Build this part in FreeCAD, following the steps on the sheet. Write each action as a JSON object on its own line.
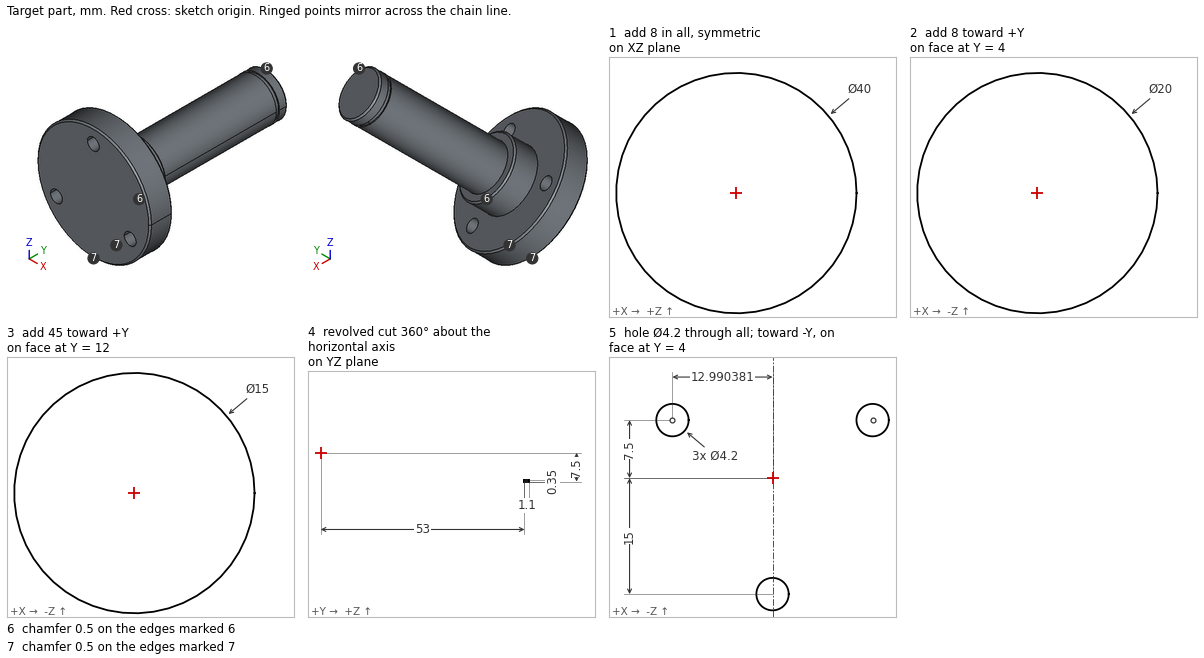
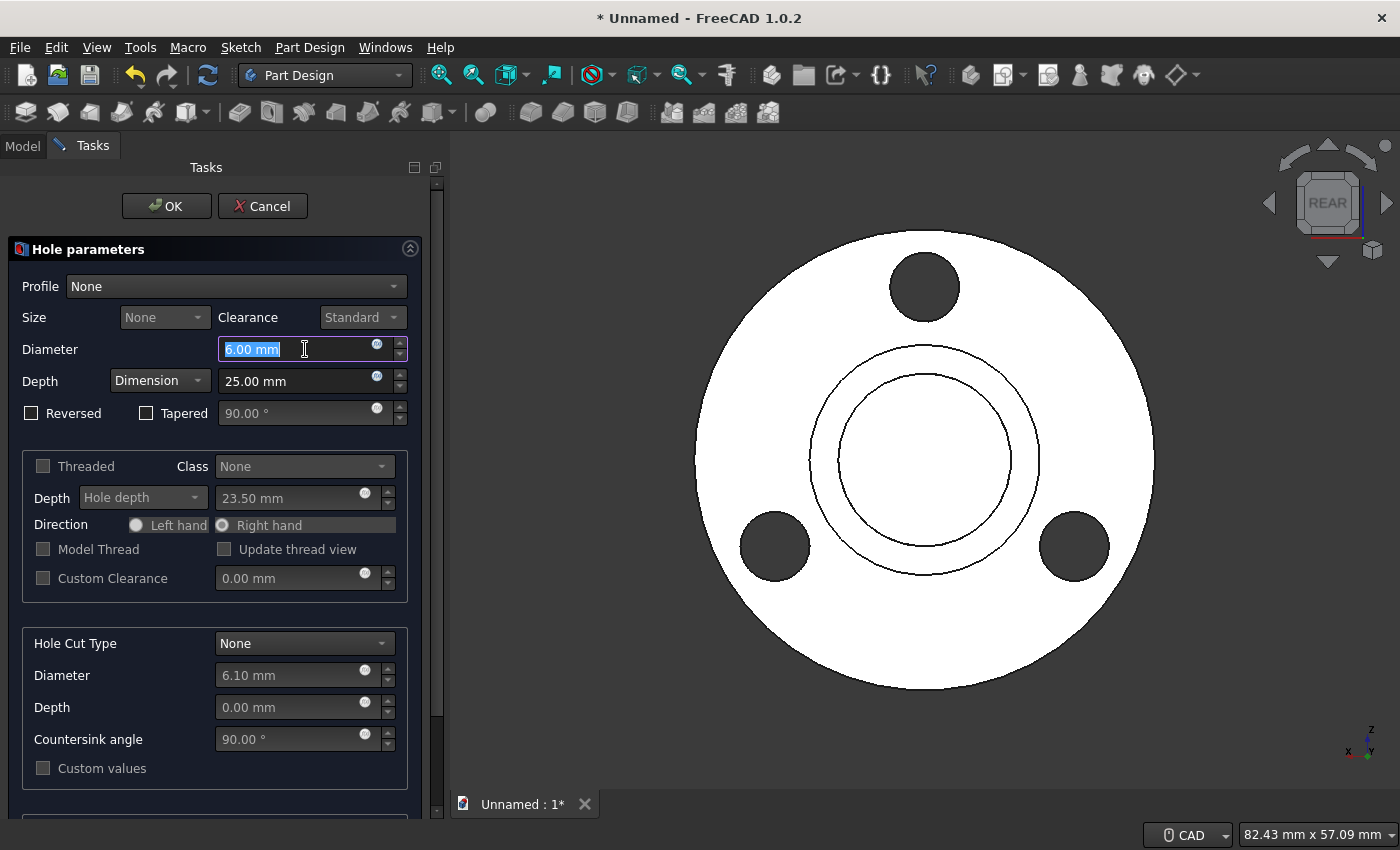
{"action": "type", "text": "4.2"}
{"action": "key", "text": "Tab"}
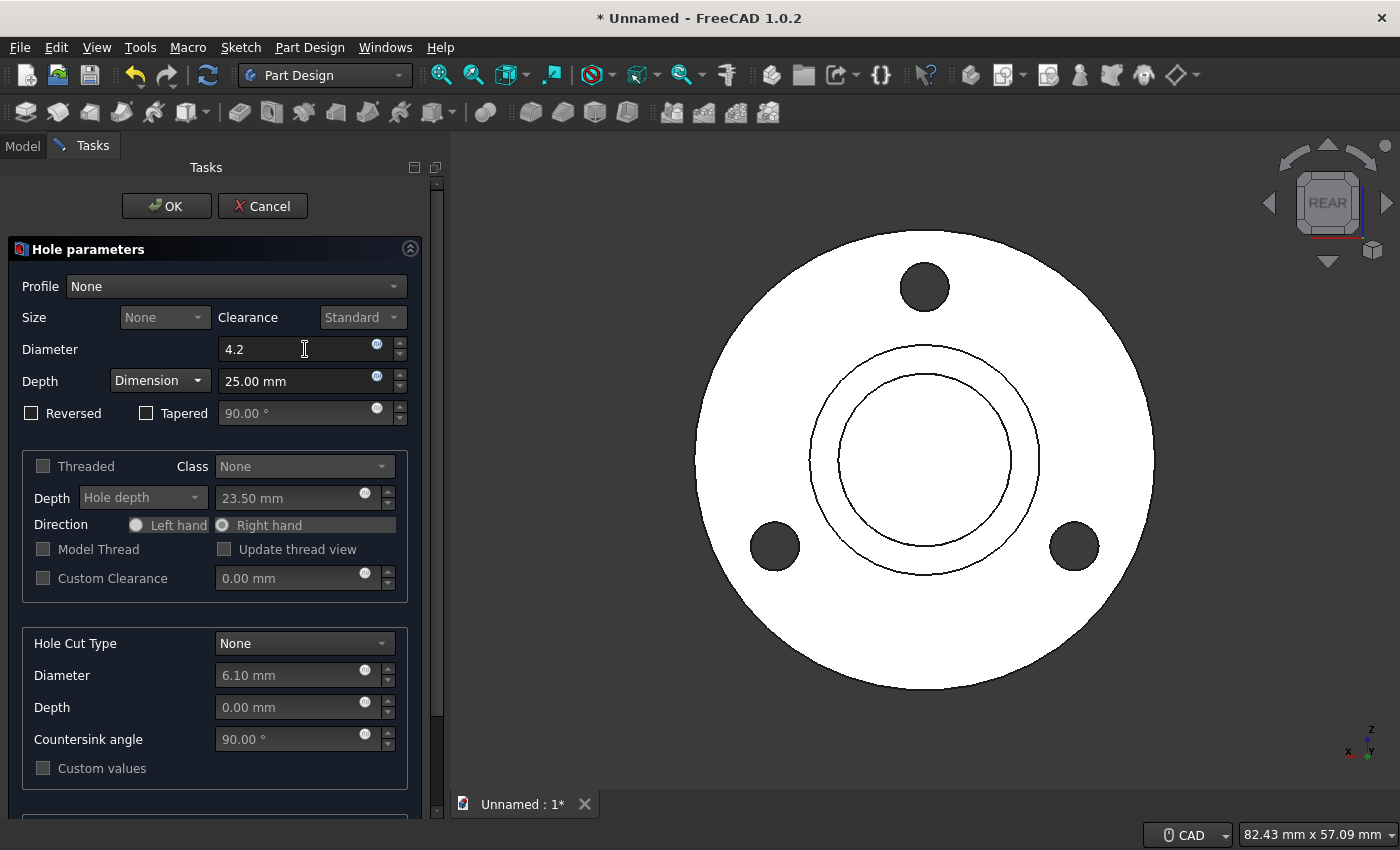
{"action": "left_click", "coordinate": [161, 380]}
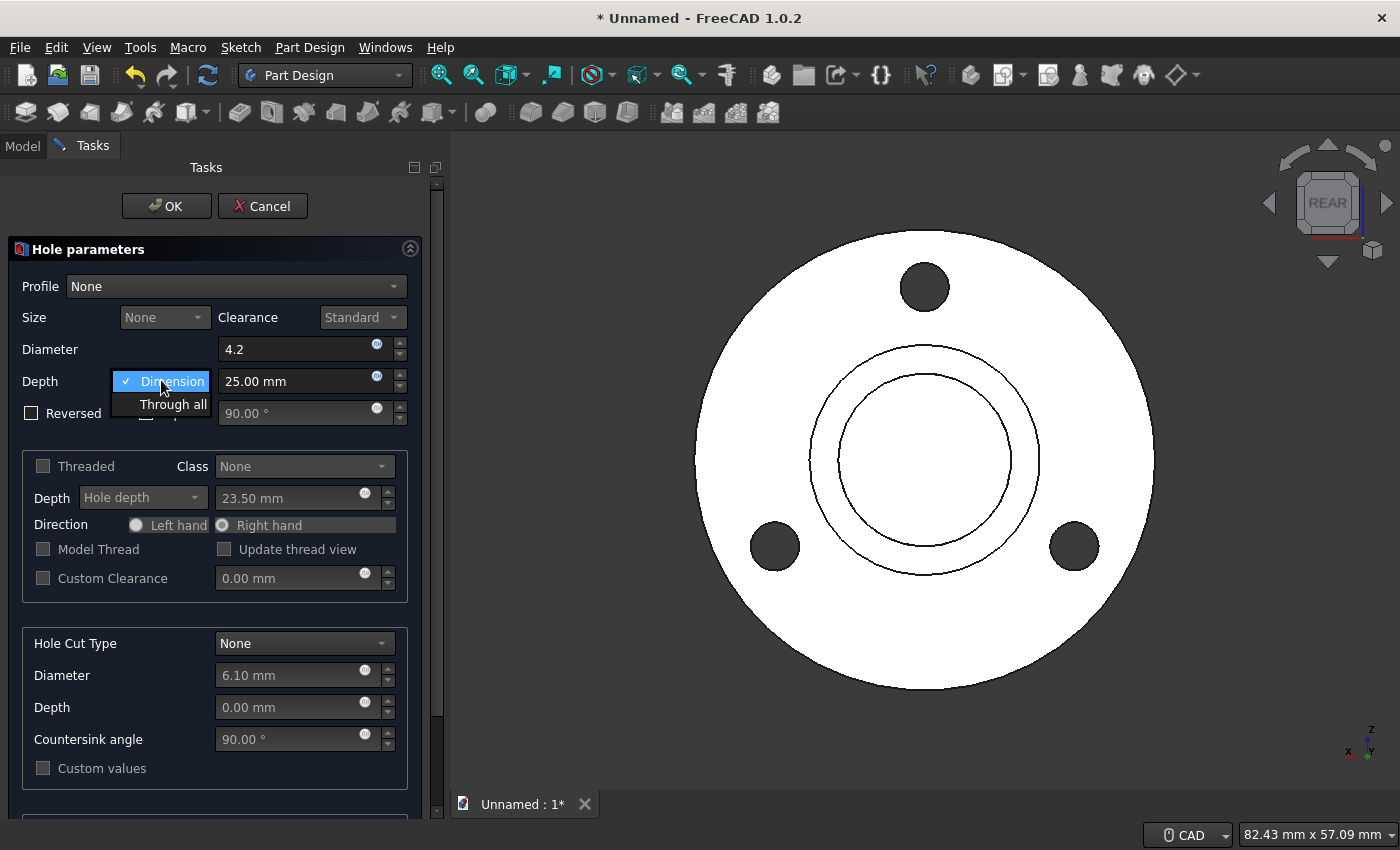
{"action": "left_click", "coordinate": [160, 404]}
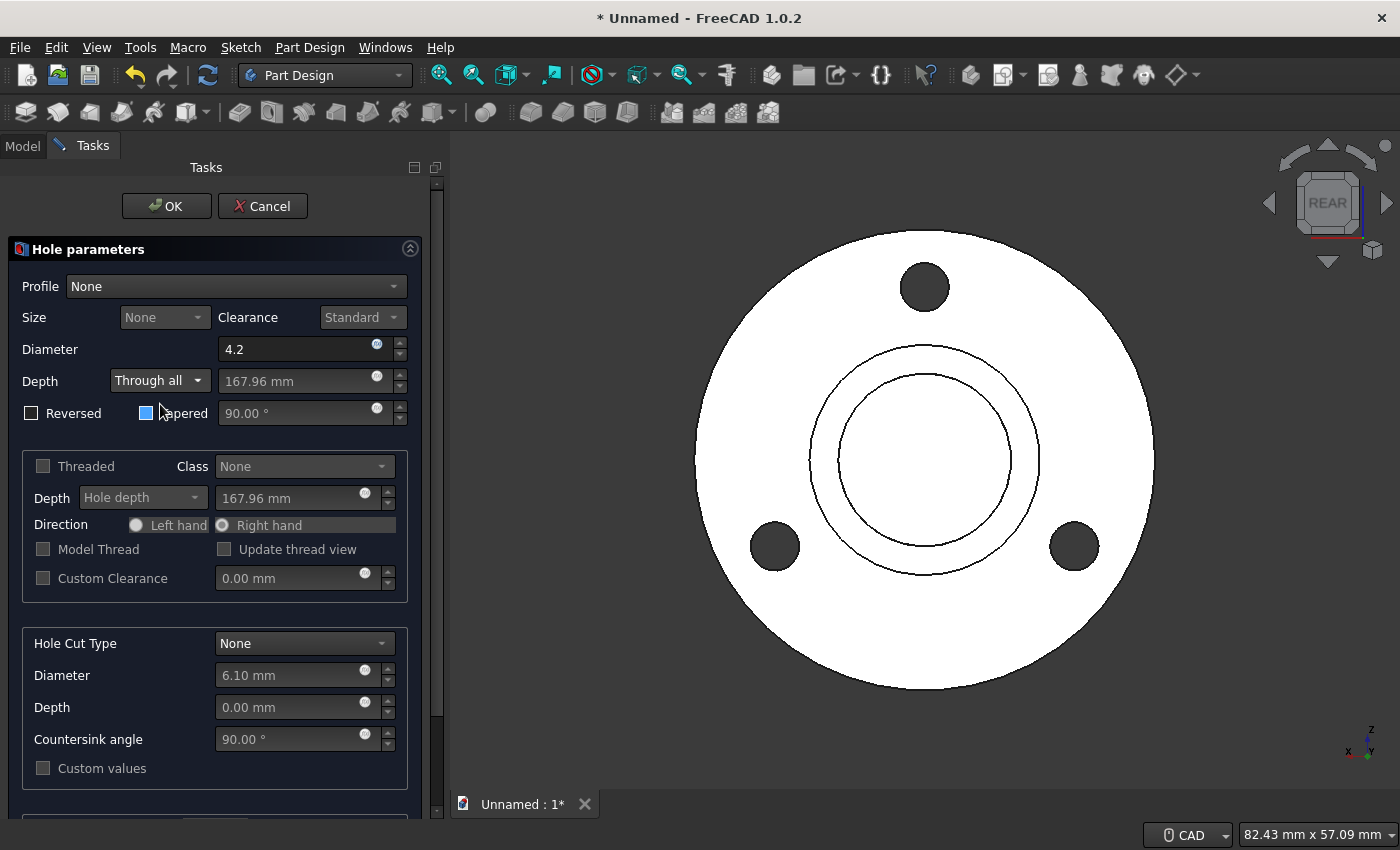
{"action": "left_click", "coordinate": [167, 206]}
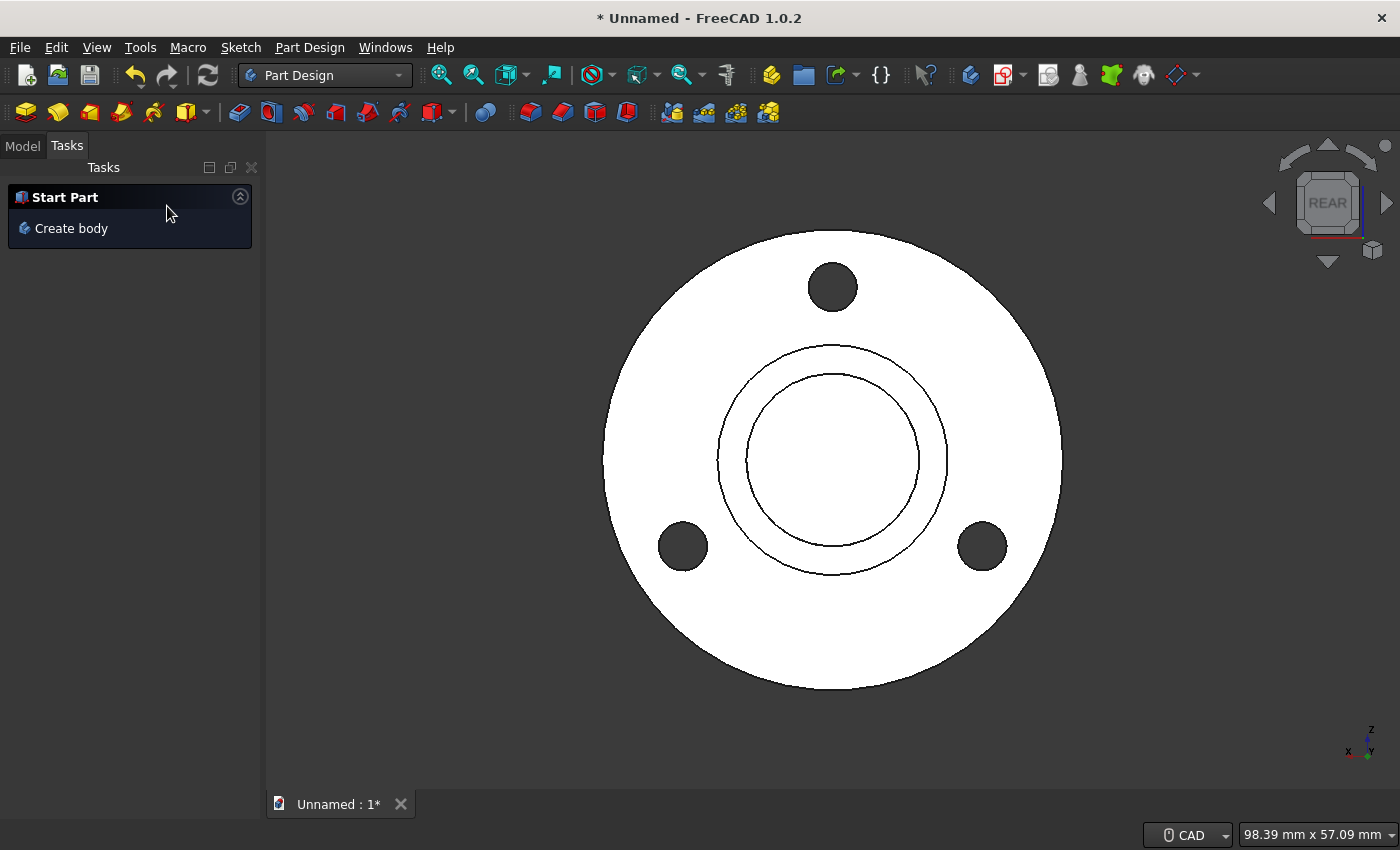
{"action": "left_click", "coordinate": [919, 459]}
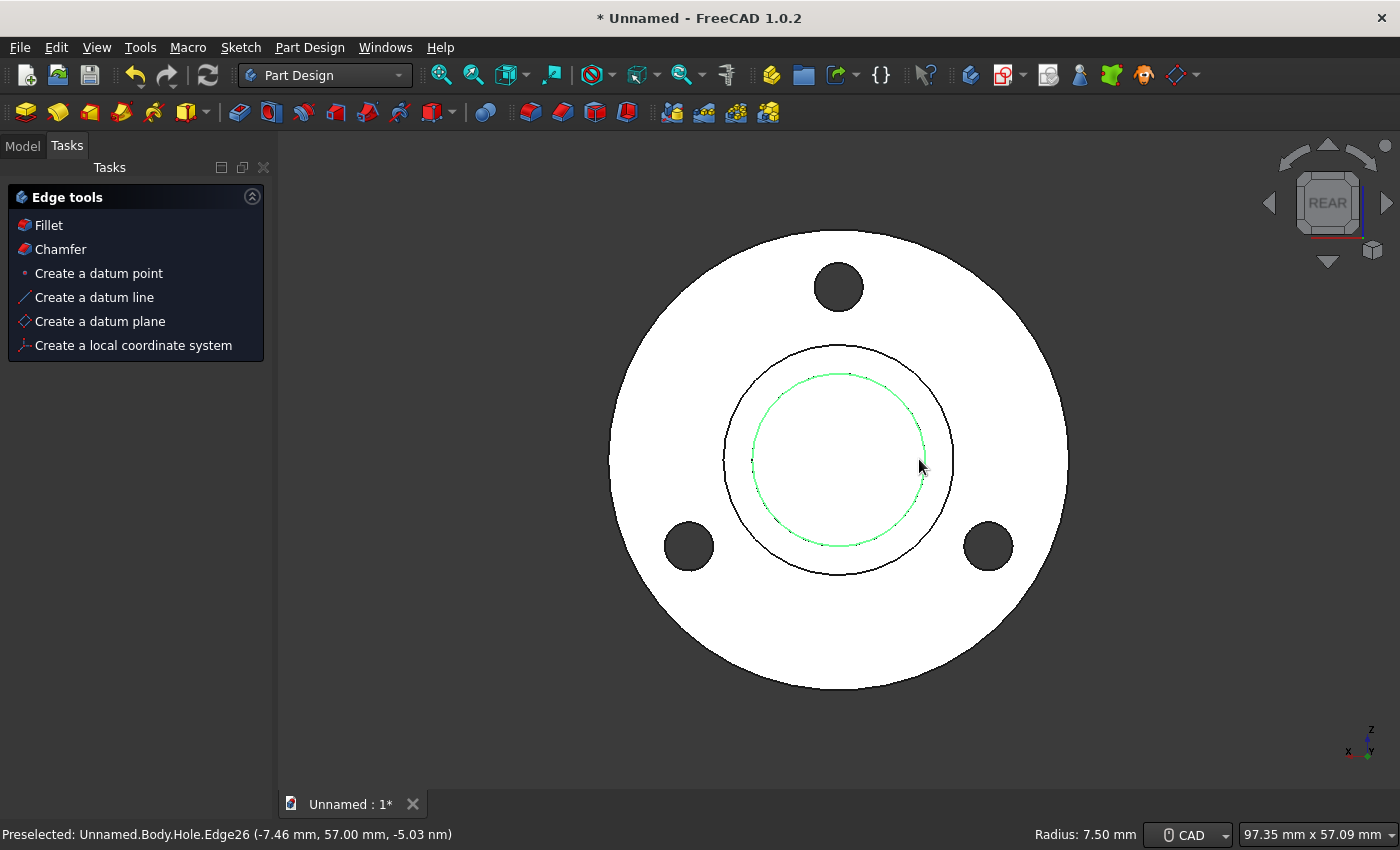
{"action": "left_click", "coordinate": [954, 459], "text": "ctrl"}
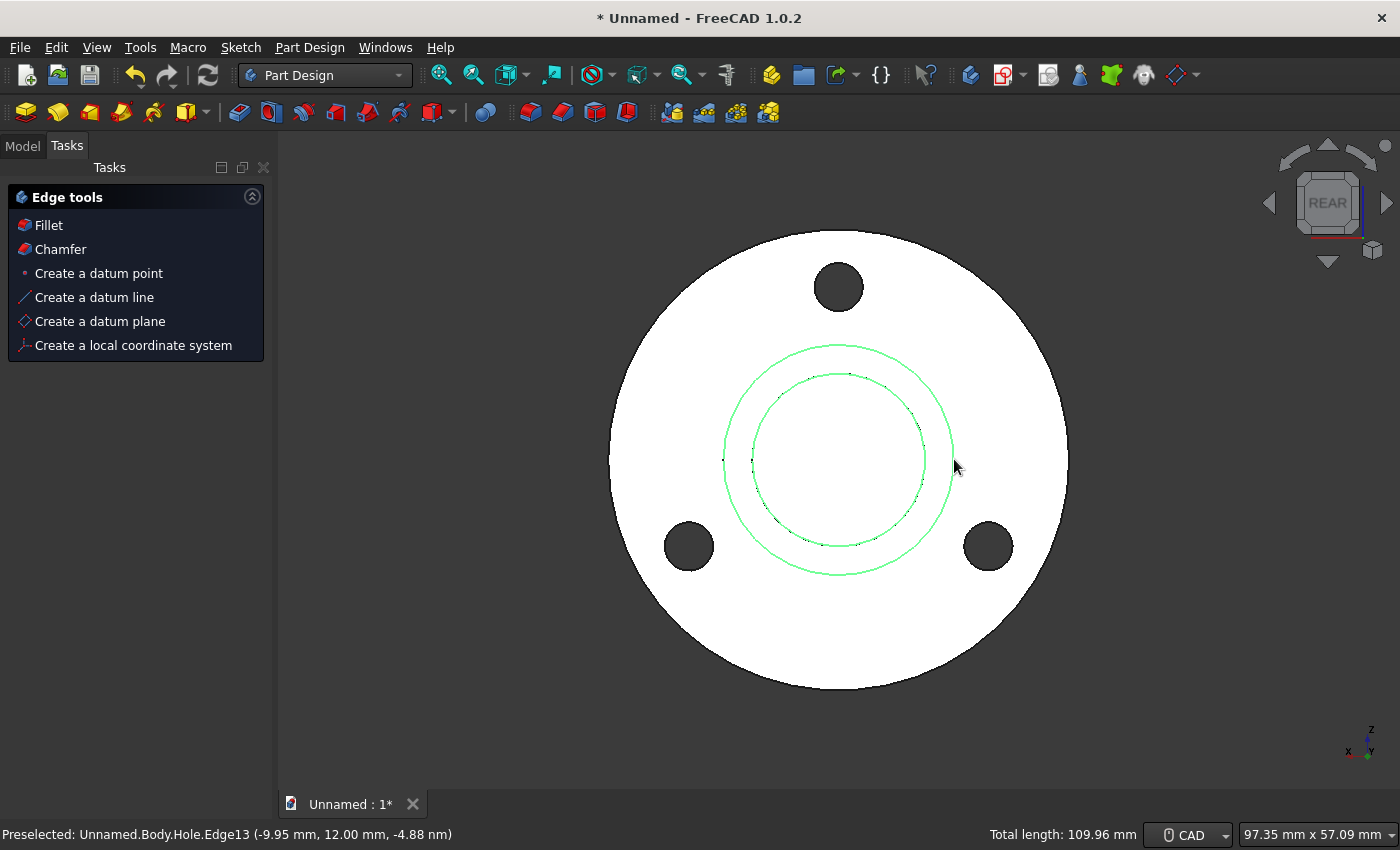
{"action": "left_click", "coordinate": [564, 112]}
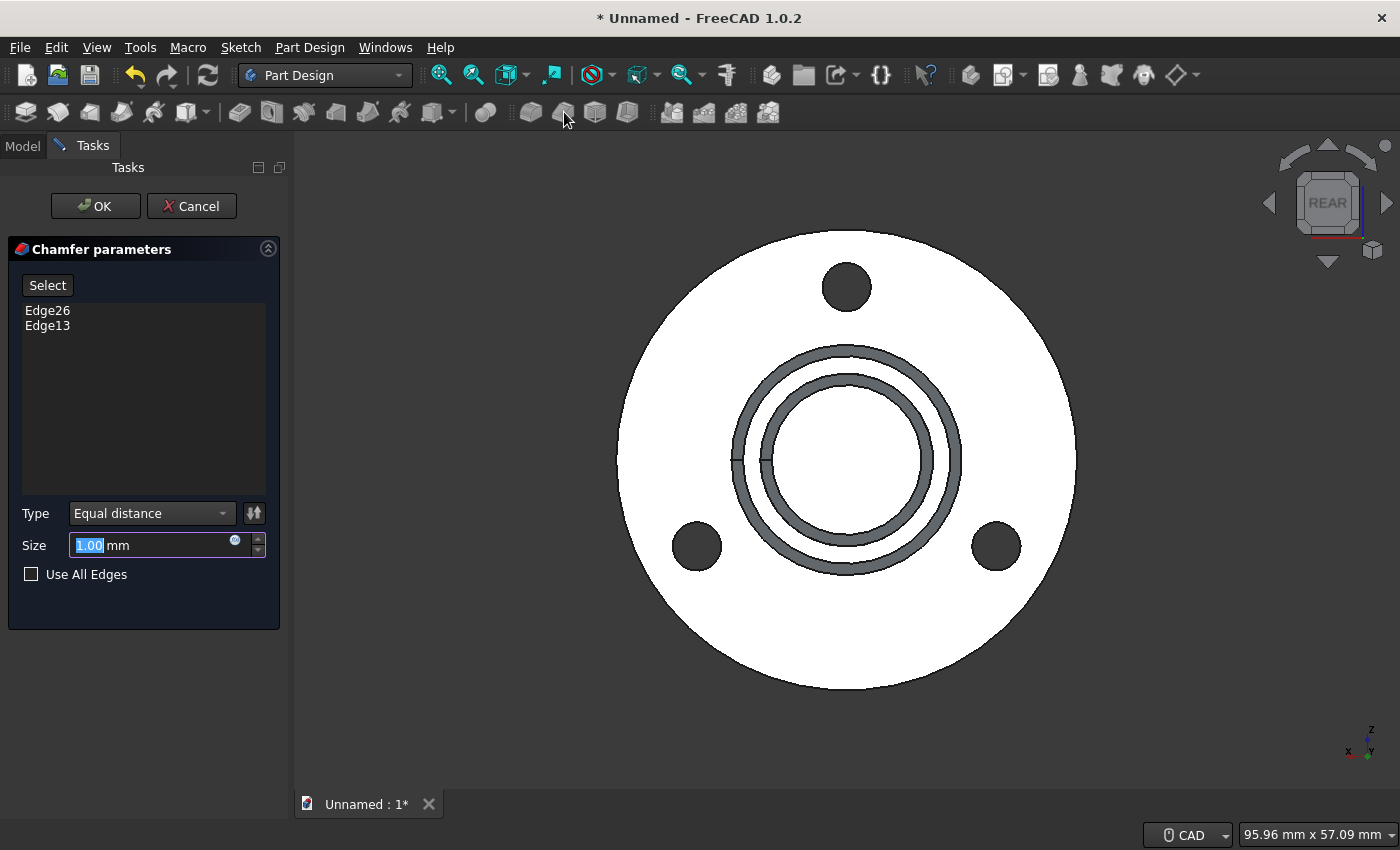
{"action": "type", "text": "0.5"}
{"action": "key", "text": "Tab"}